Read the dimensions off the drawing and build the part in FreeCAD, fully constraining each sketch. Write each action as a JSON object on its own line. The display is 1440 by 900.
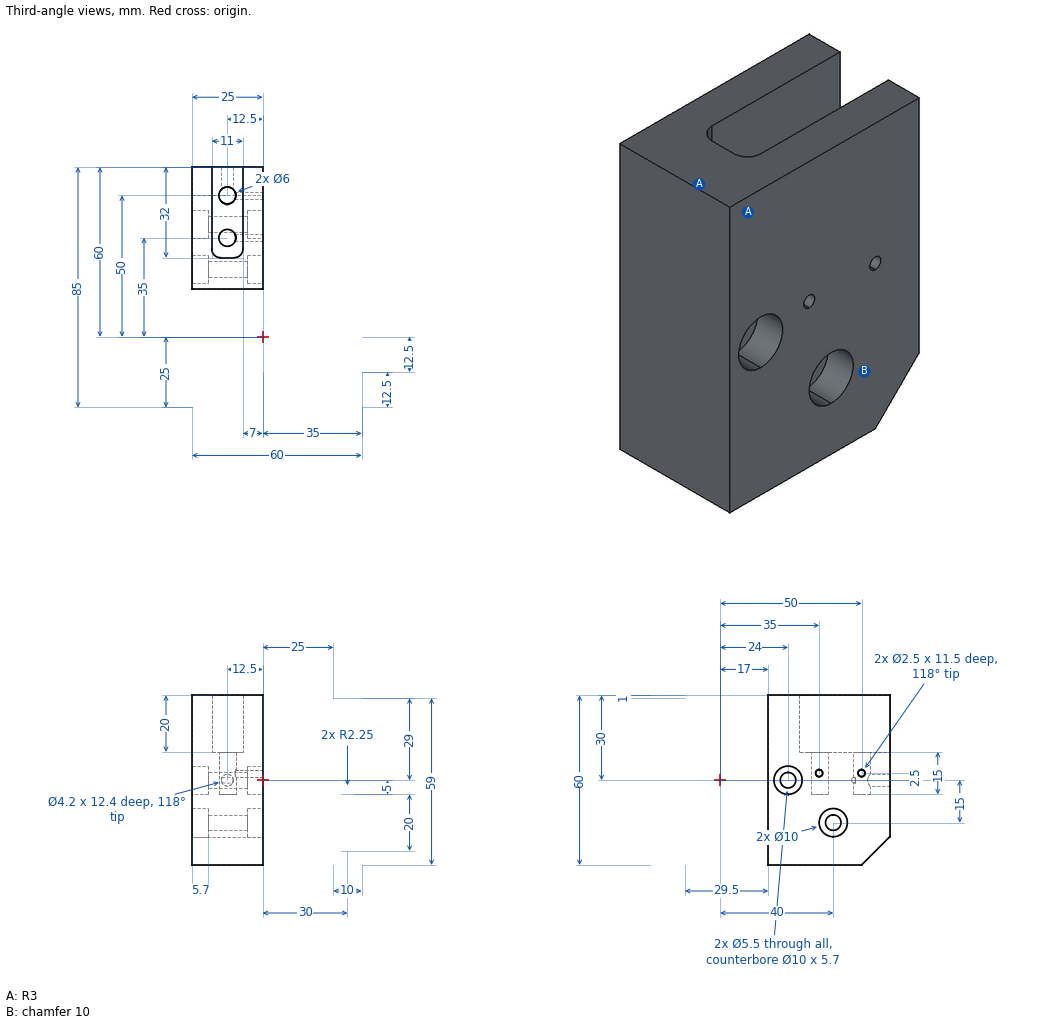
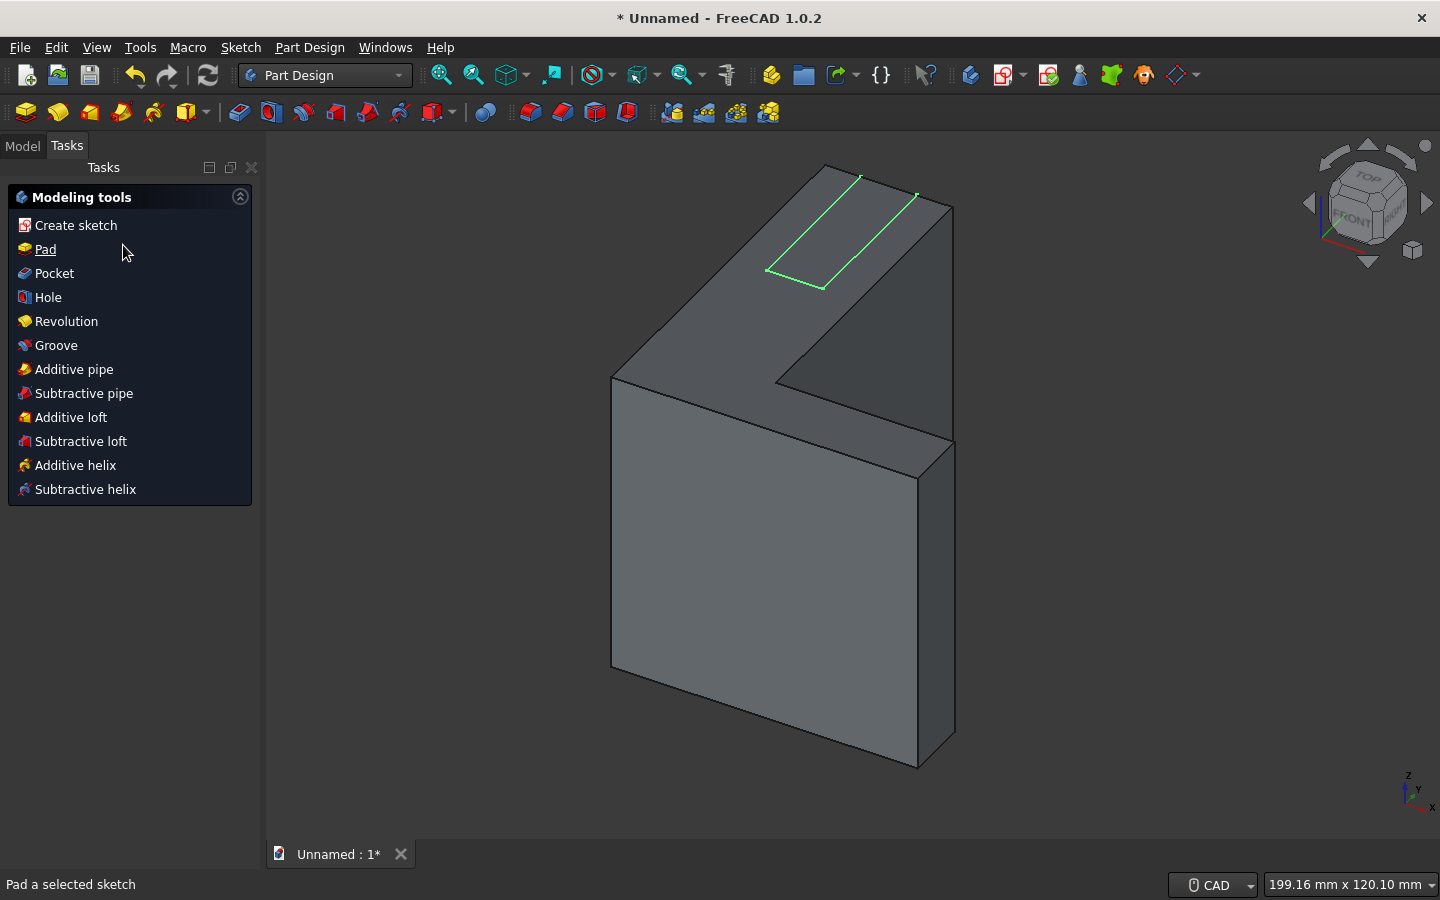
{"action": "left_click", "coordinate": [240, 112]}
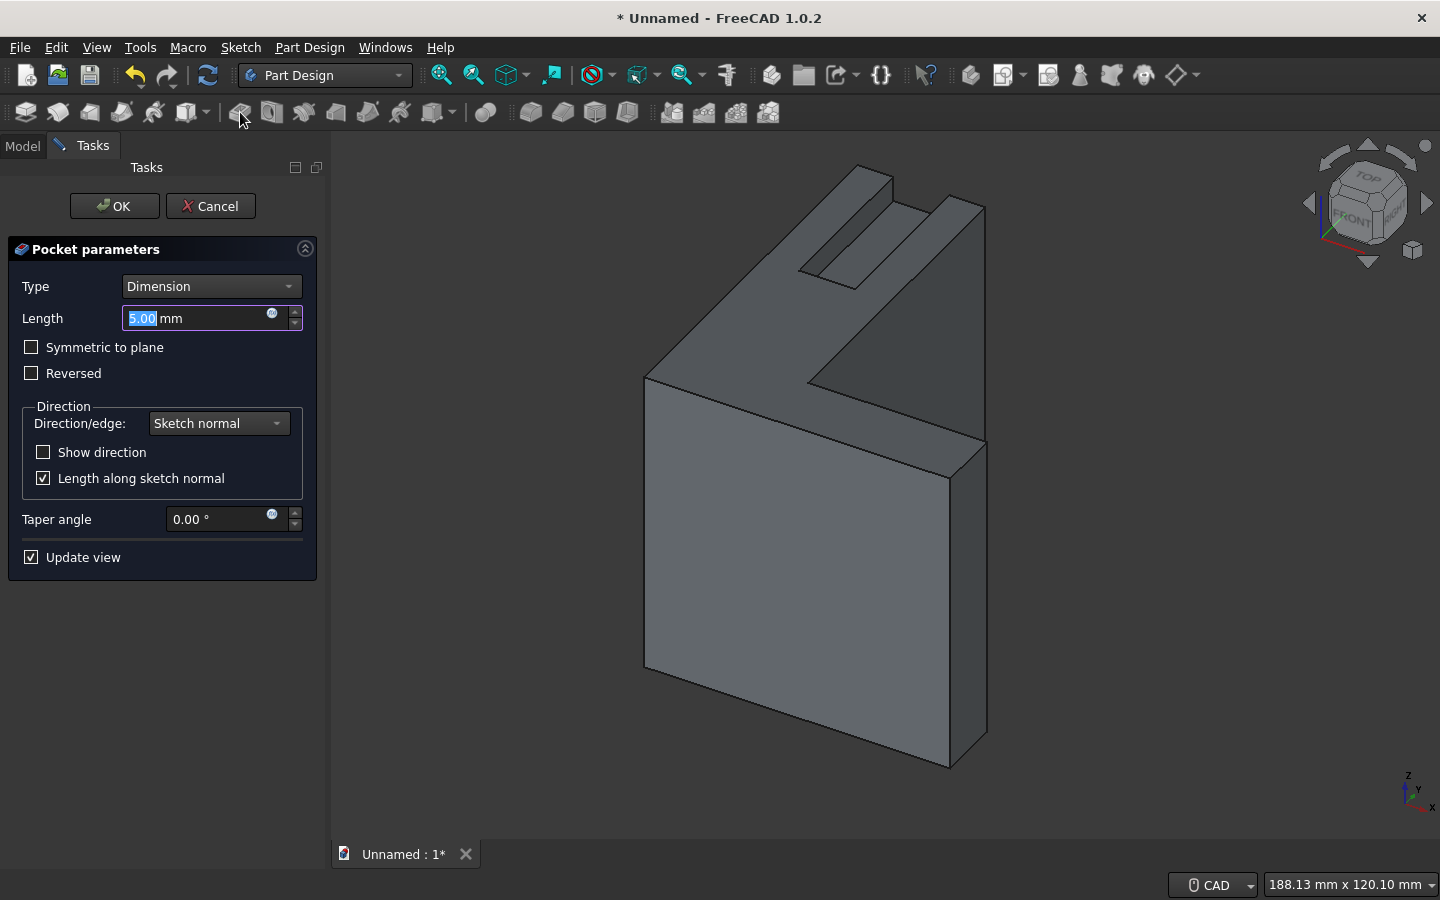
{"action": "type", "text": "20"}
{"action": "key", "text": "Tab"}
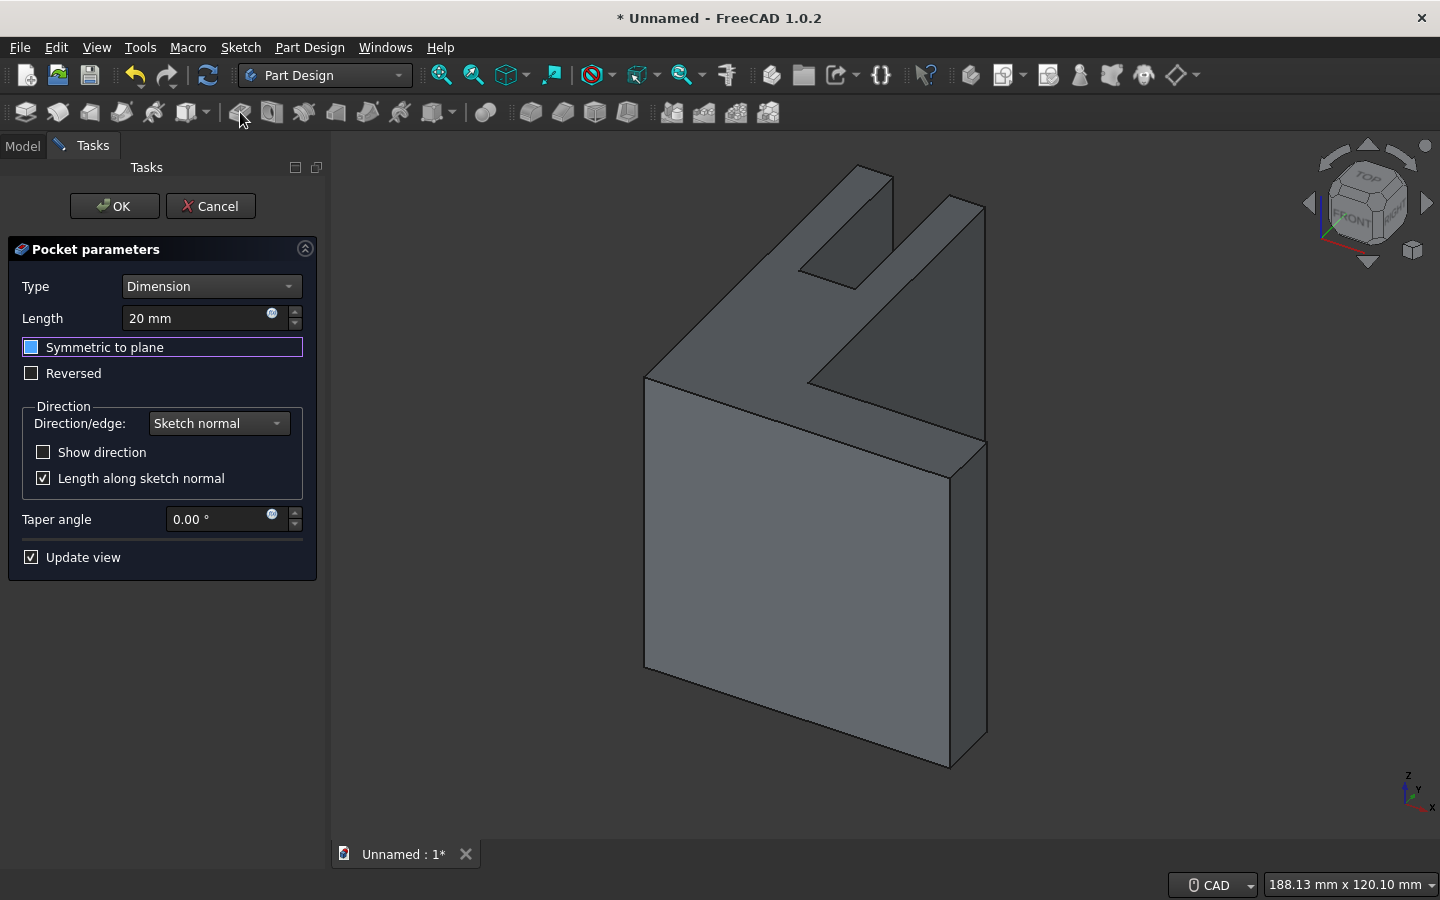
{"action": "left_click", "coordinate": [115, 206]}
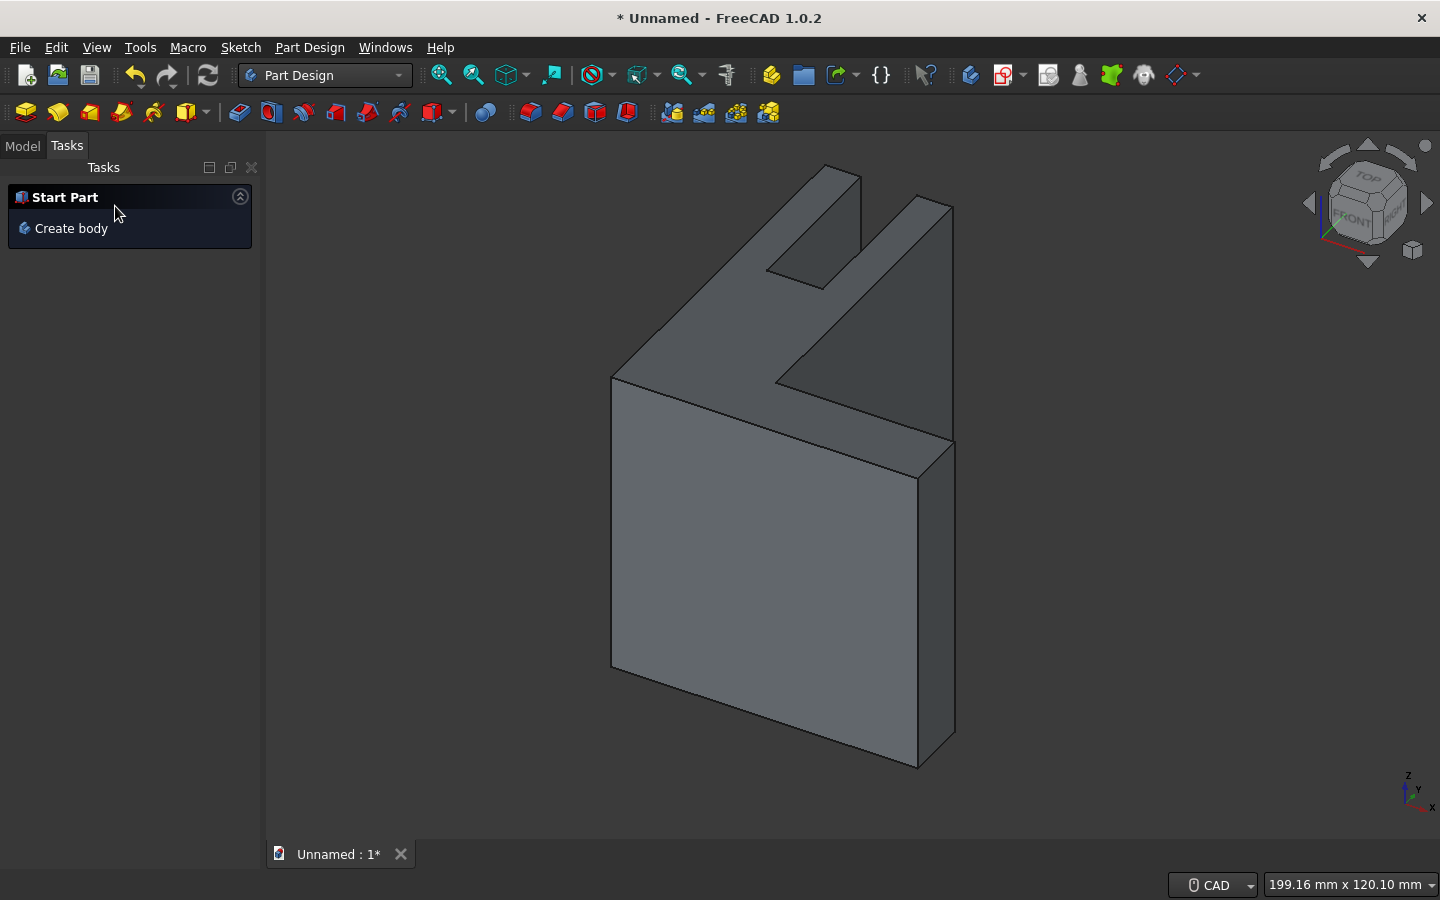
{"action": "key", "text": "0"}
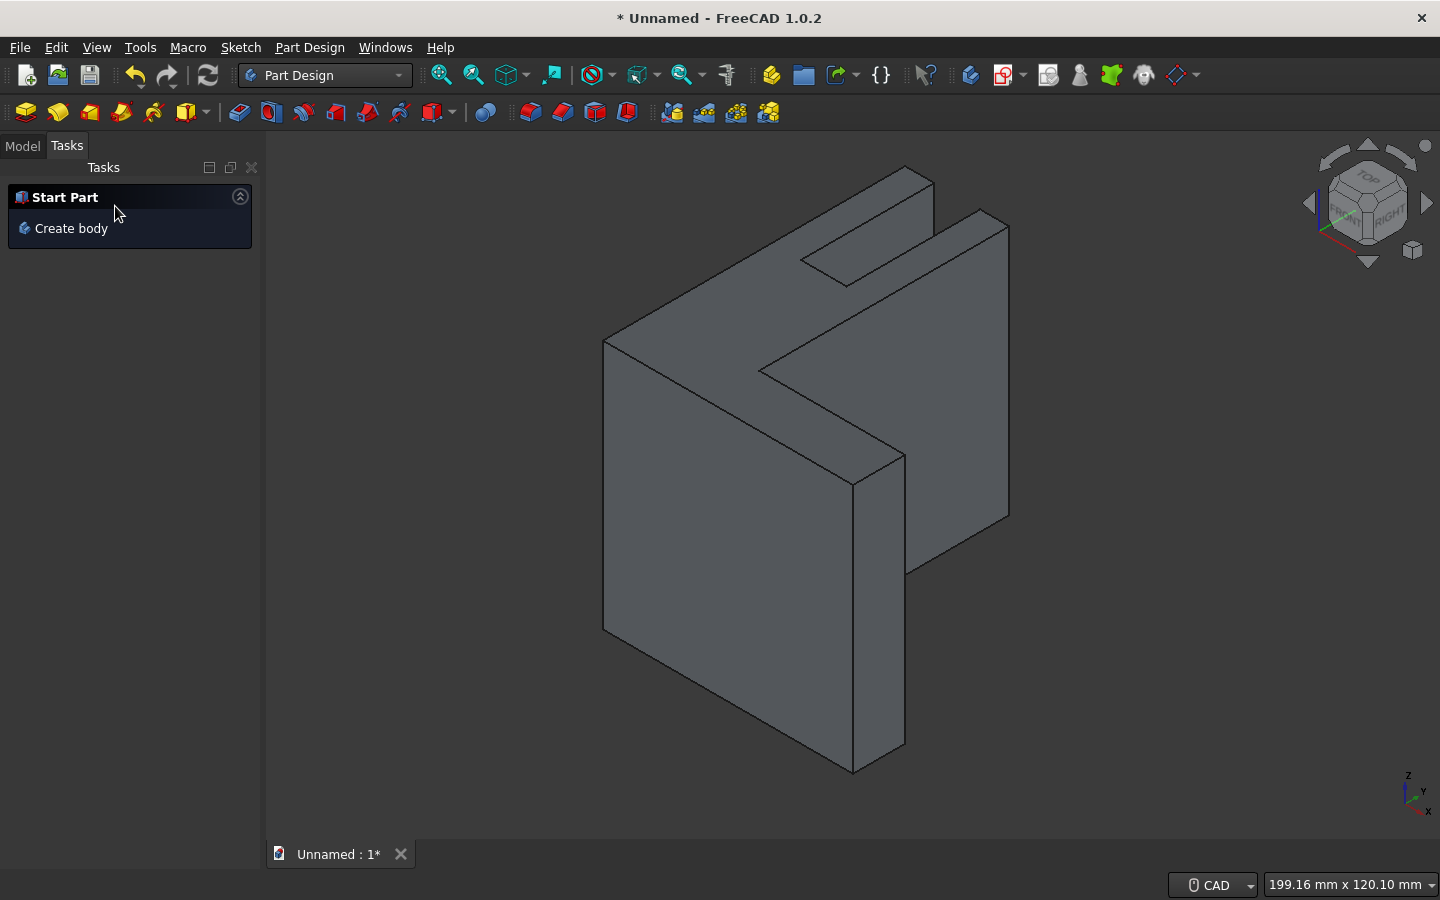
{"action": "key", "text": "2"}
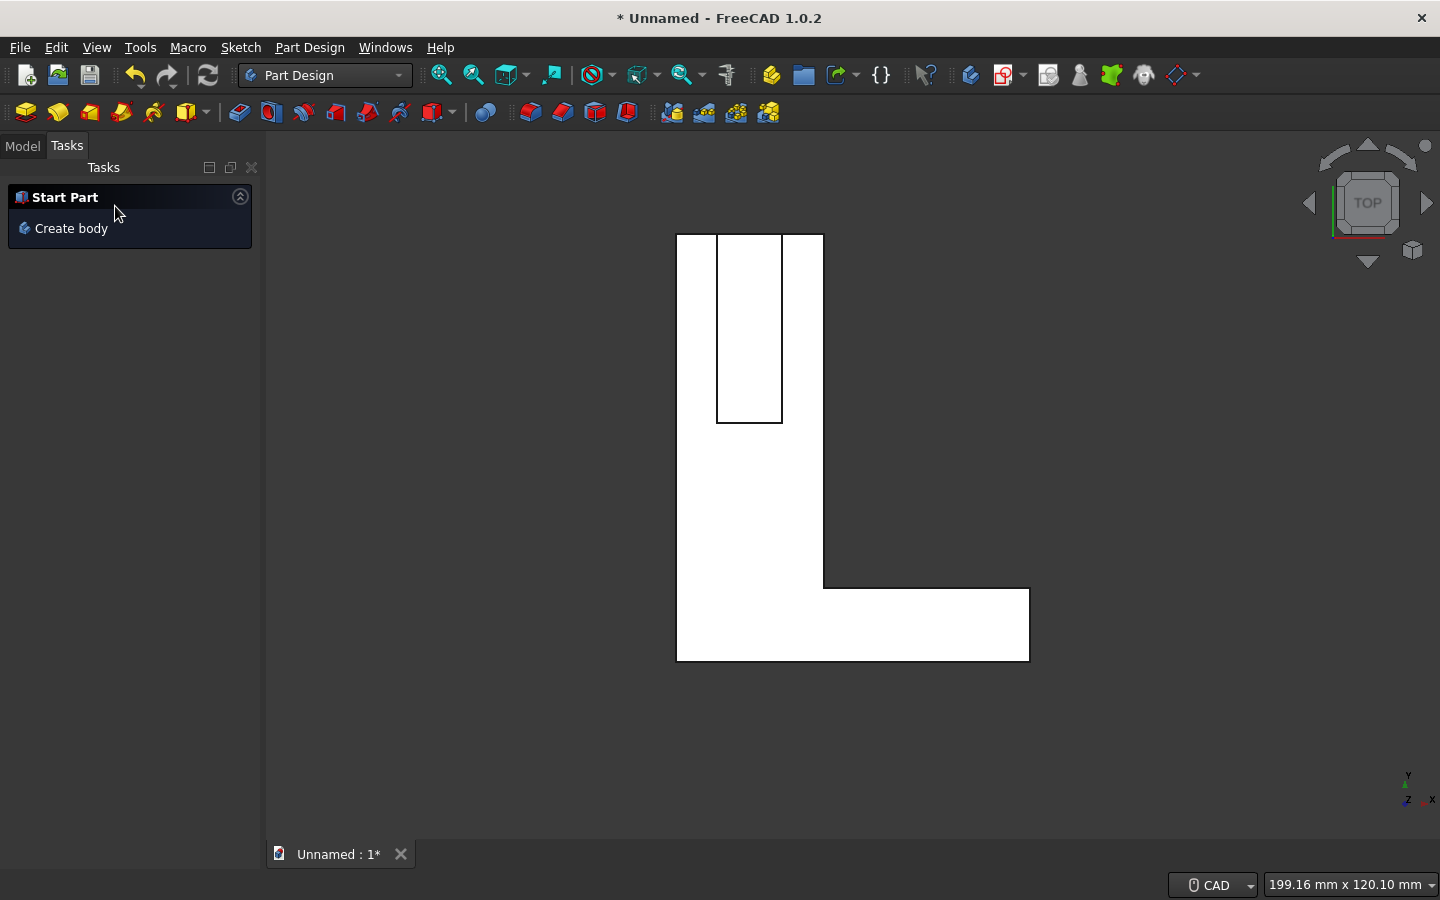
{"action": "key", "text": "1"}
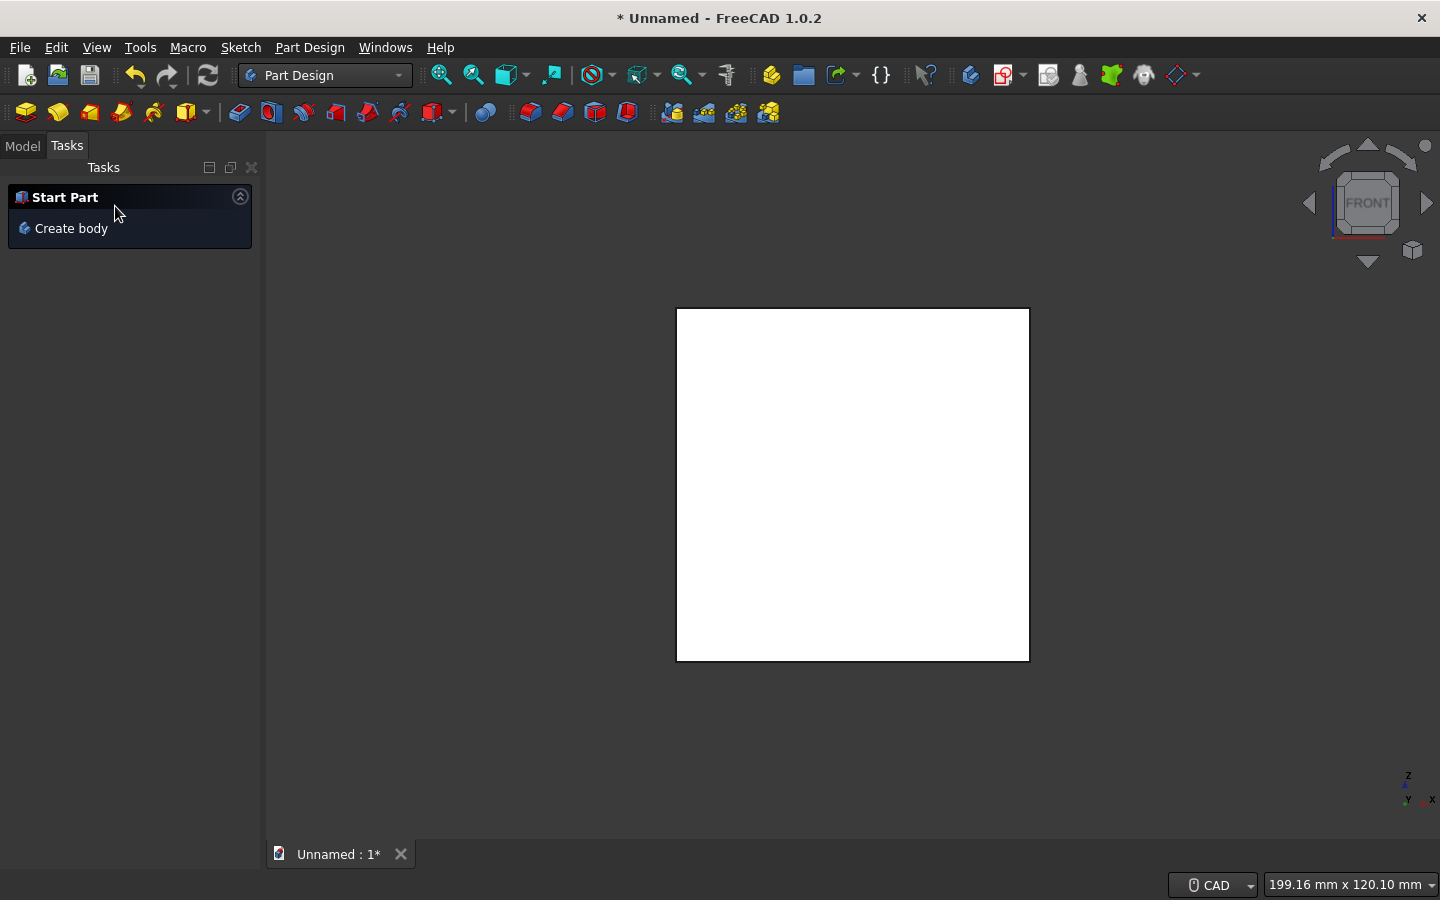
{"action": "key", "text": "3"}